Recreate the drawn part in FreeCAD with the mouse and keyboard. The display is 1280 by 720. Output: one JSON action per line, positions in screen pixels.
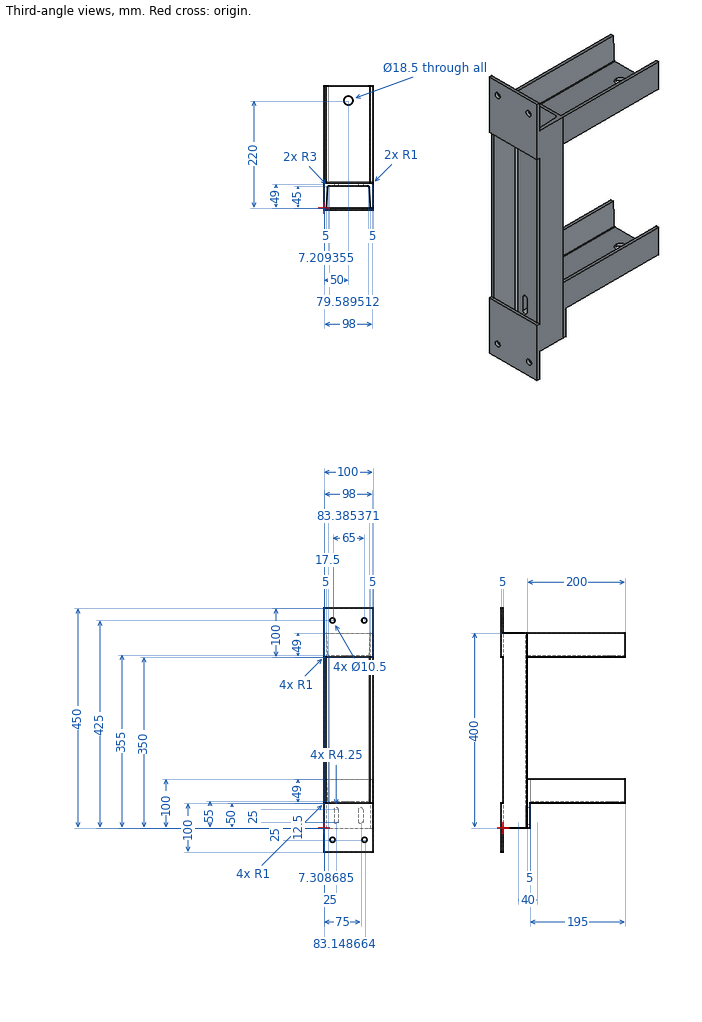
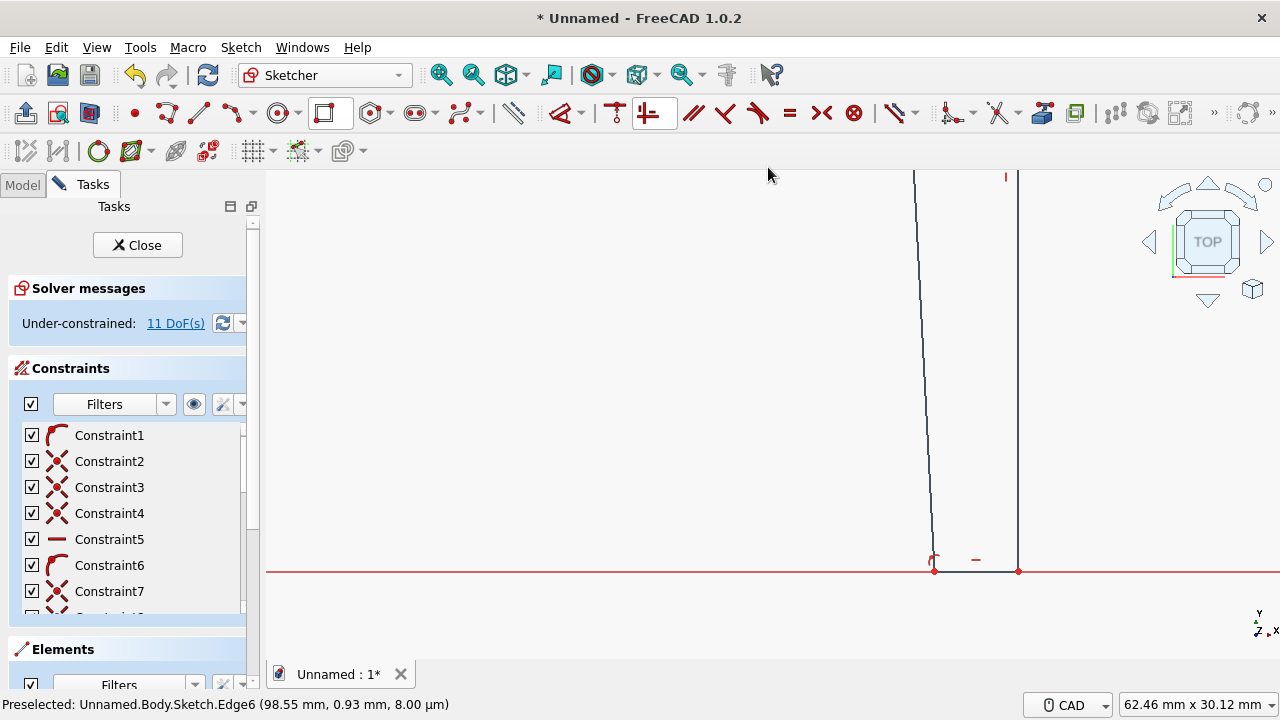
{"action": "scroll", "coordinate": [995, 559], "scroll_direction": "down", "scroll_amount": 5}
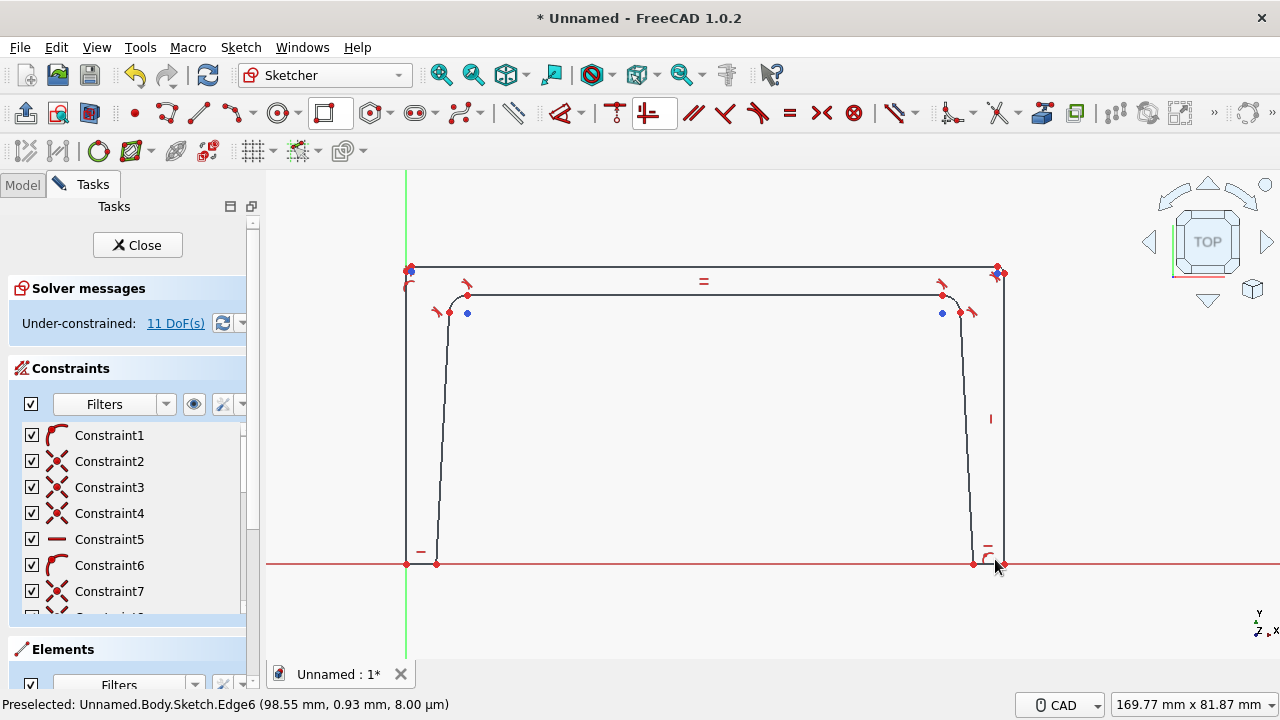
{"action": "scroll", "coordinate": [459, 297], "scroll_direction": "up", "scroll_amount": 3}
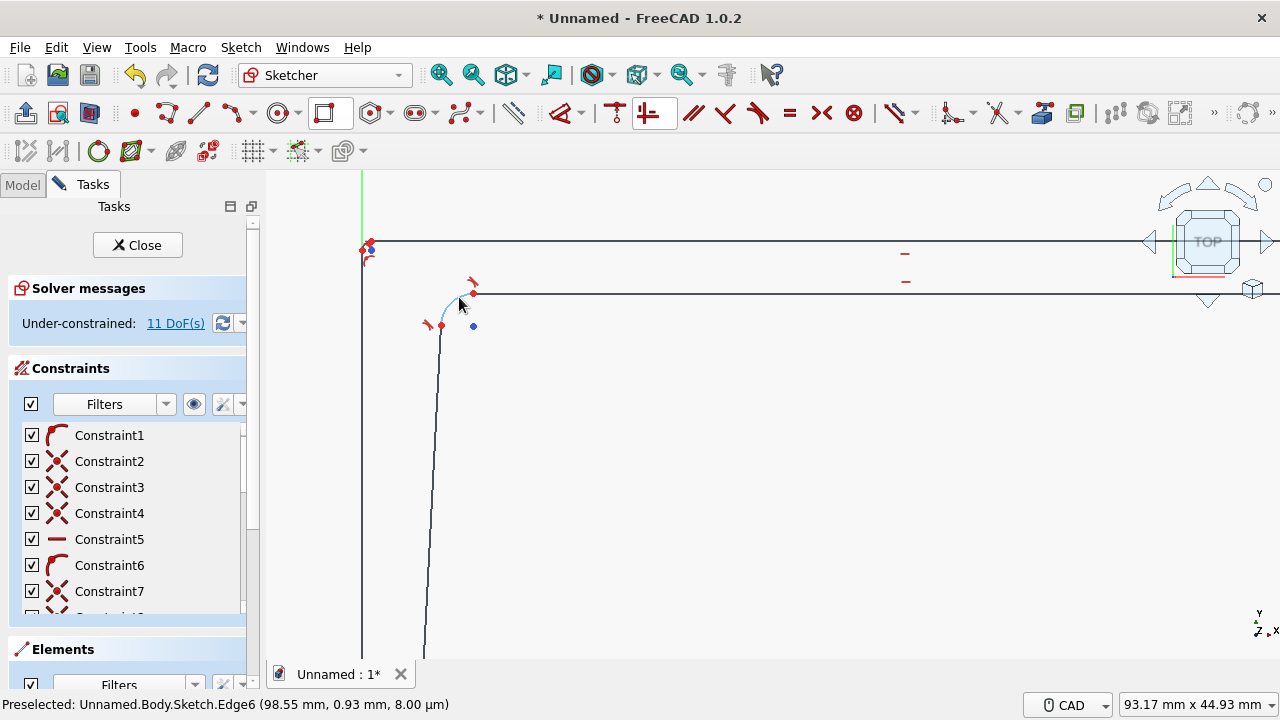
{"action": "left_click", "coordinate": [459, 297]}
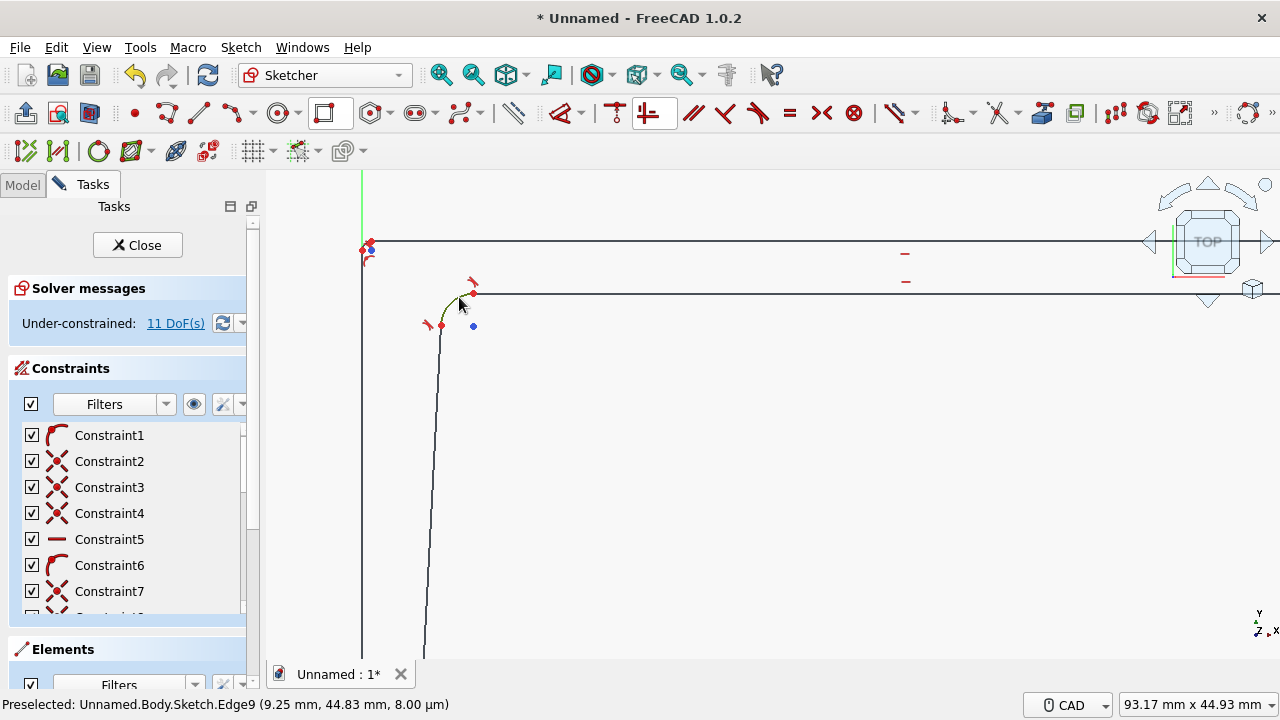
{"action": "scroll", "coordinate": [459, 297], "scroll_direction": "down", "scroll_amount": 3}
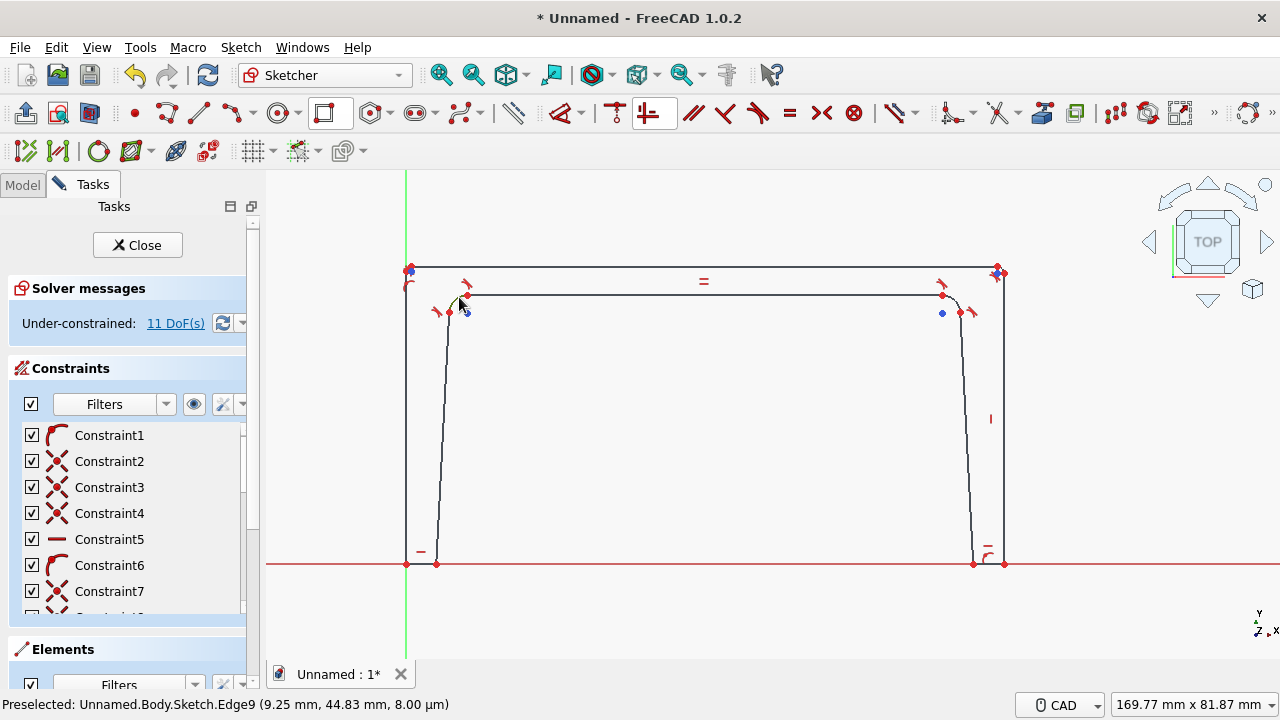
{"action": "scroll", "coordinate": [958, 305], "scroll_direction": "up", "scroll_amount": 3}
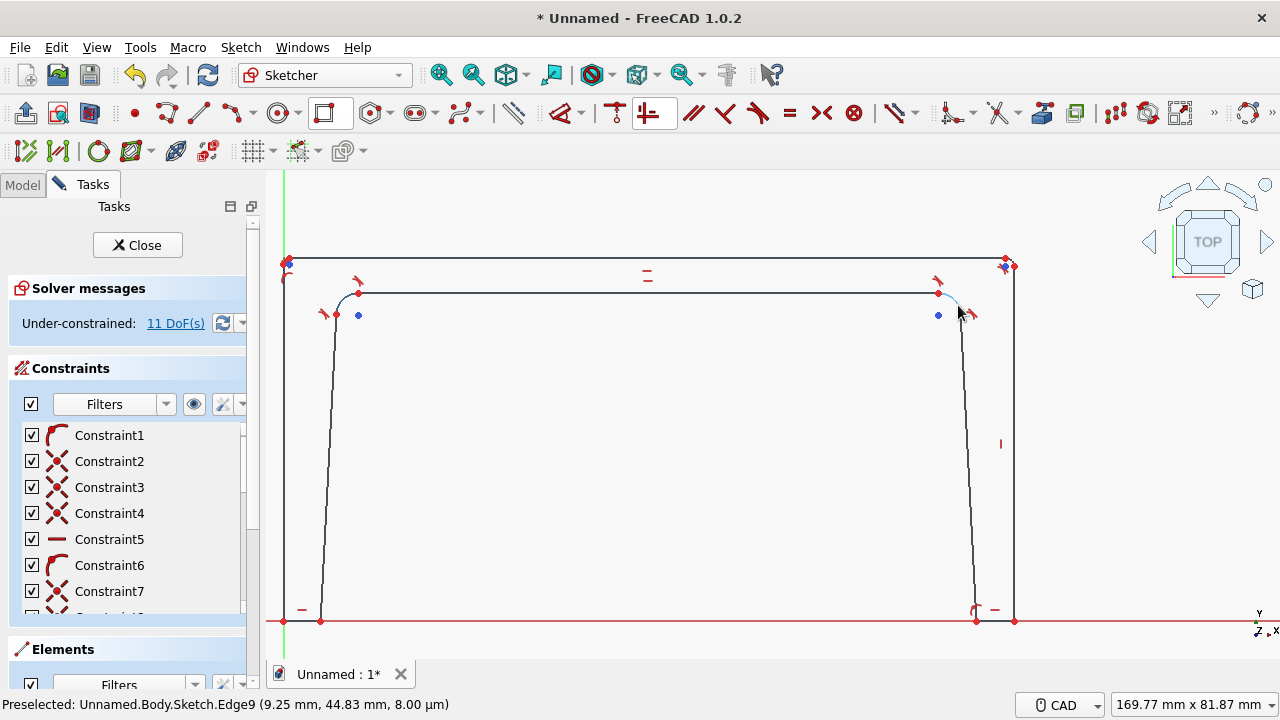
{"action": "left_click", "coordinate": [957, 304]}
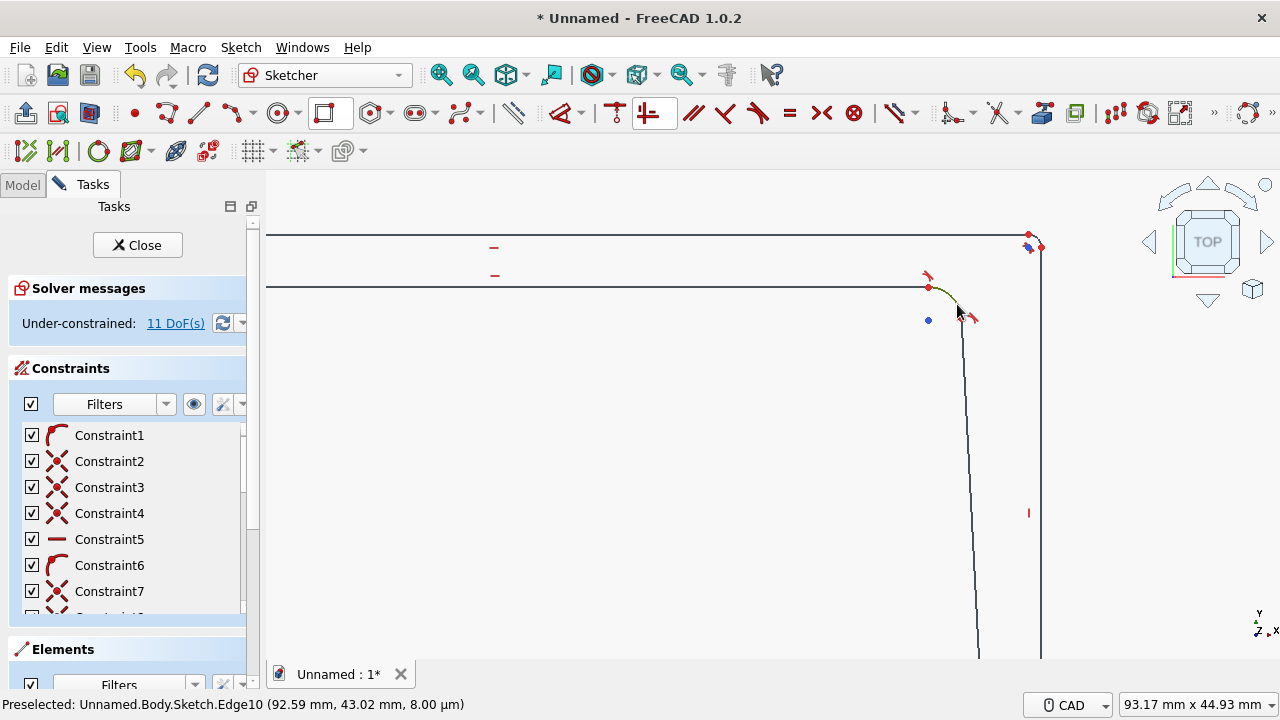
{"action": "key", "text": "e"}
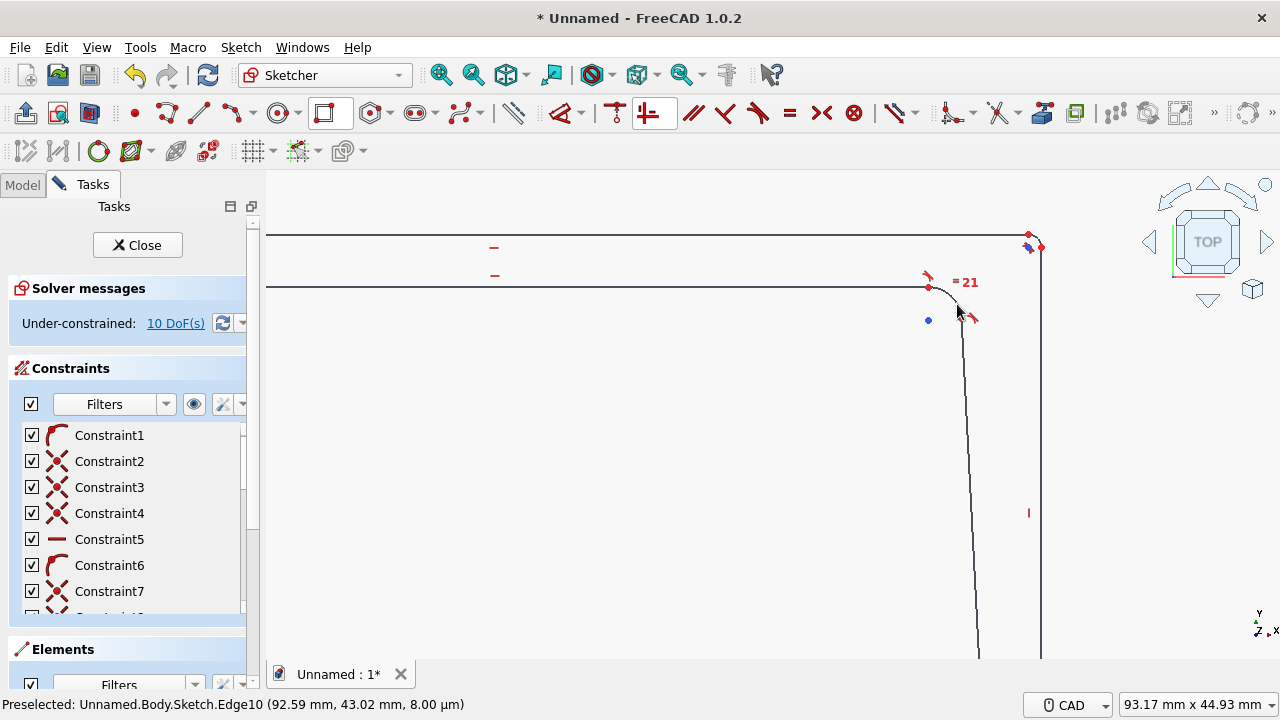
{"action": "scroll", "coordinate": [1038, 238], "scroll_direction": "up", "scroll_amount": 2}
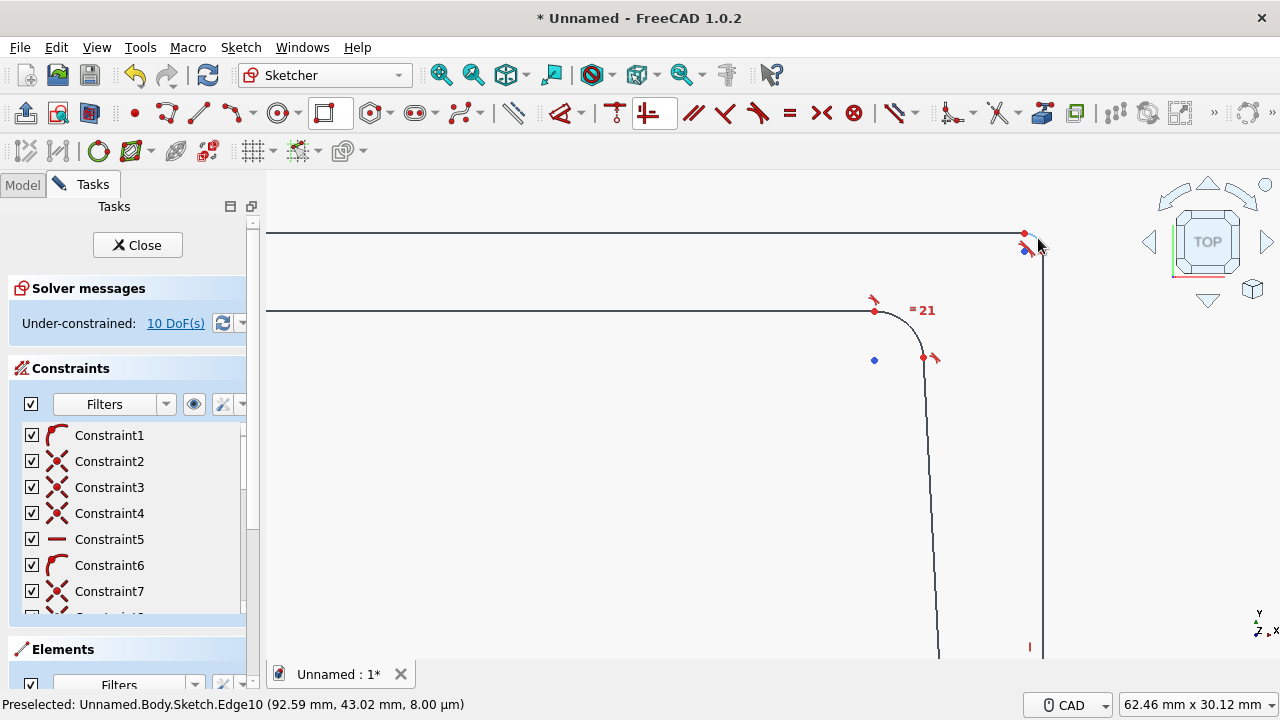
{"action": "left_click", "coordinate": [1037, 239]}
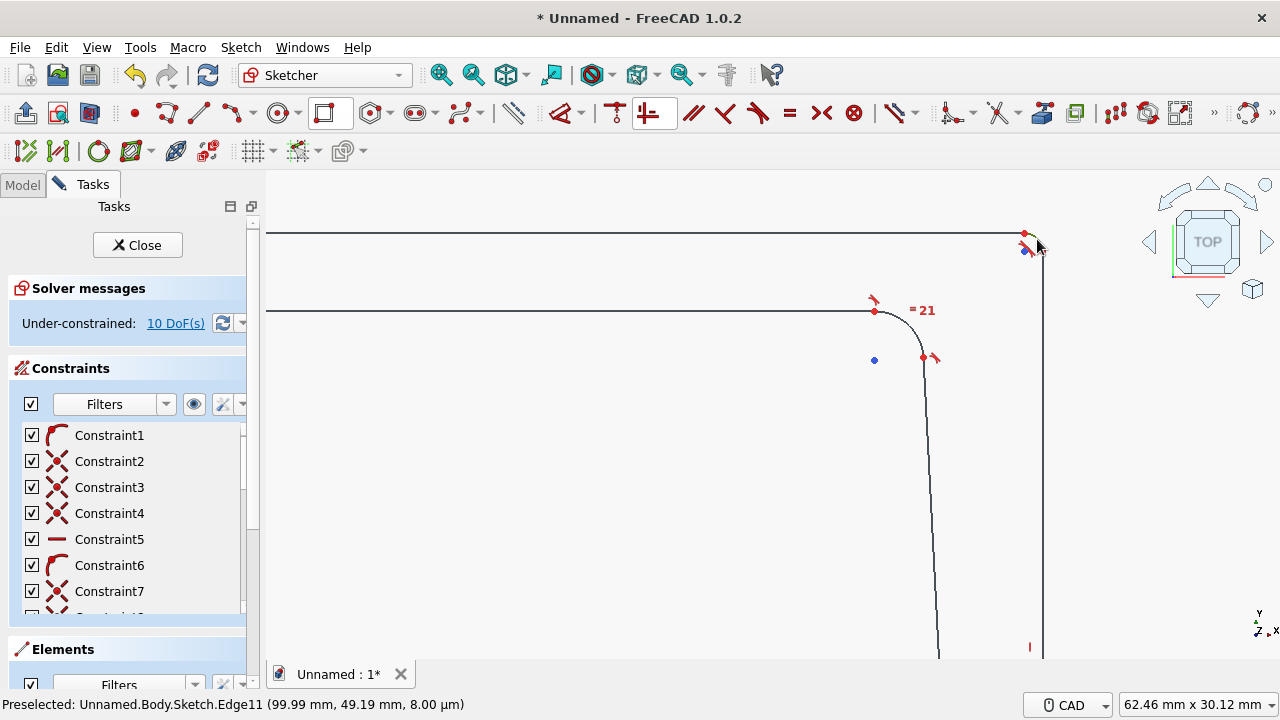
{"action": "scroll", "coordinate": [981, 286], "scroll_direction": "down", "scroll_amount": 5}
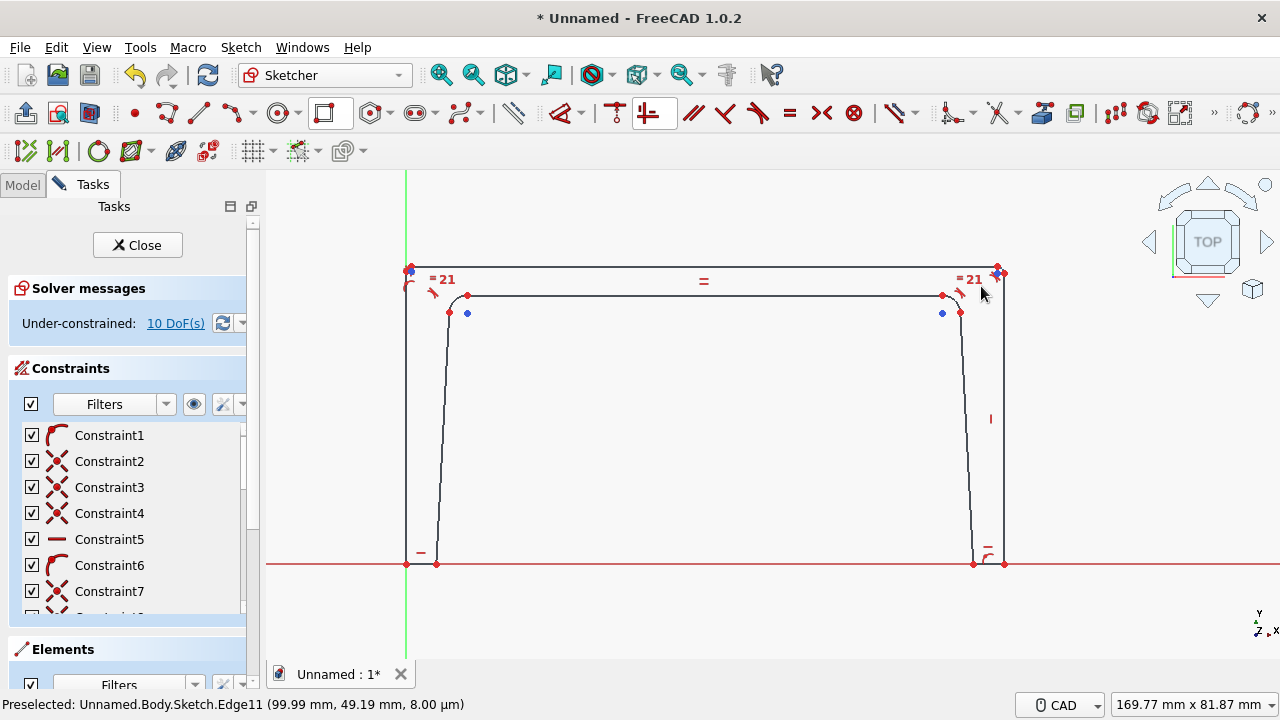
{"action": "scroll", "coordinate": [409, 267], "scroll_direction": "up", "scroll_amount": 9}